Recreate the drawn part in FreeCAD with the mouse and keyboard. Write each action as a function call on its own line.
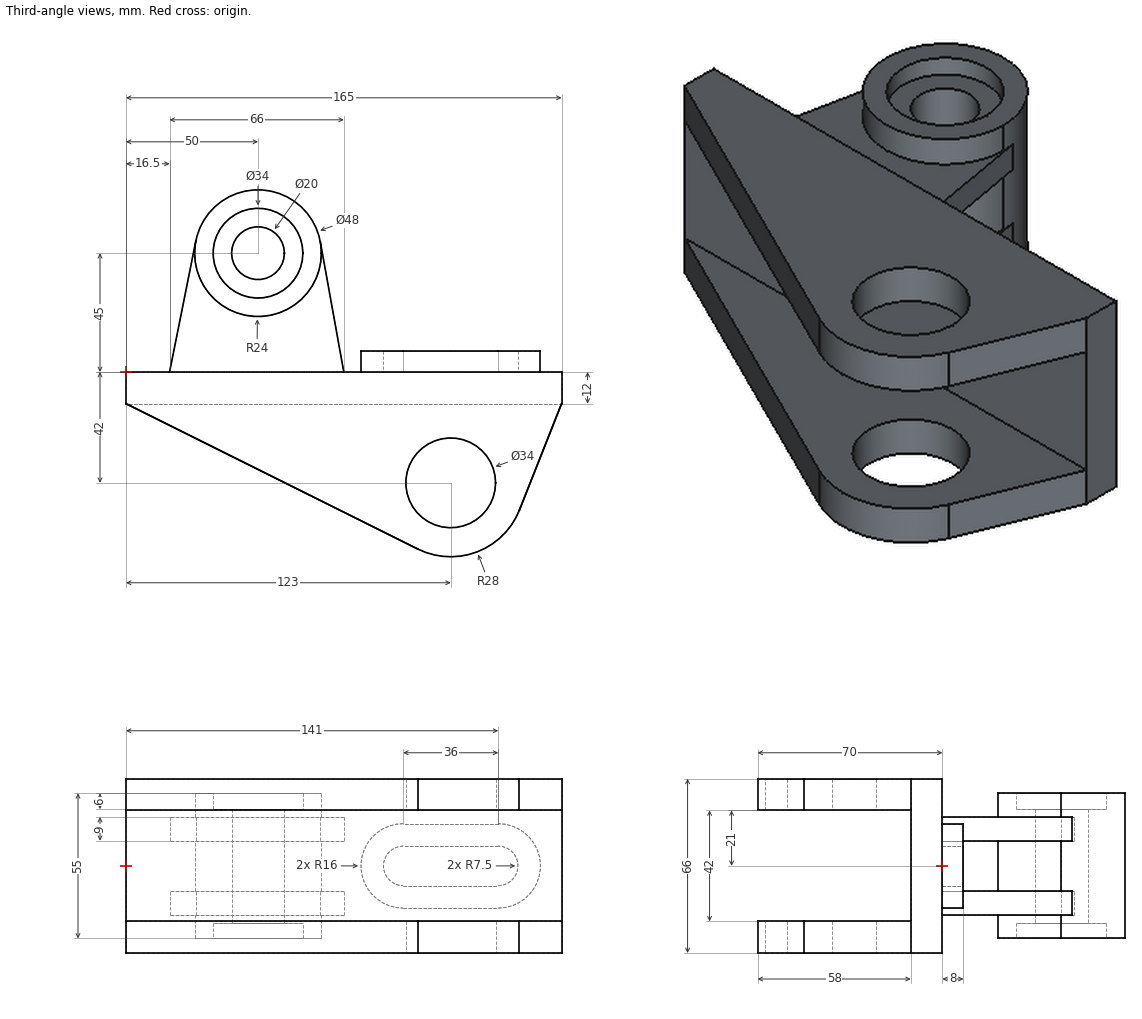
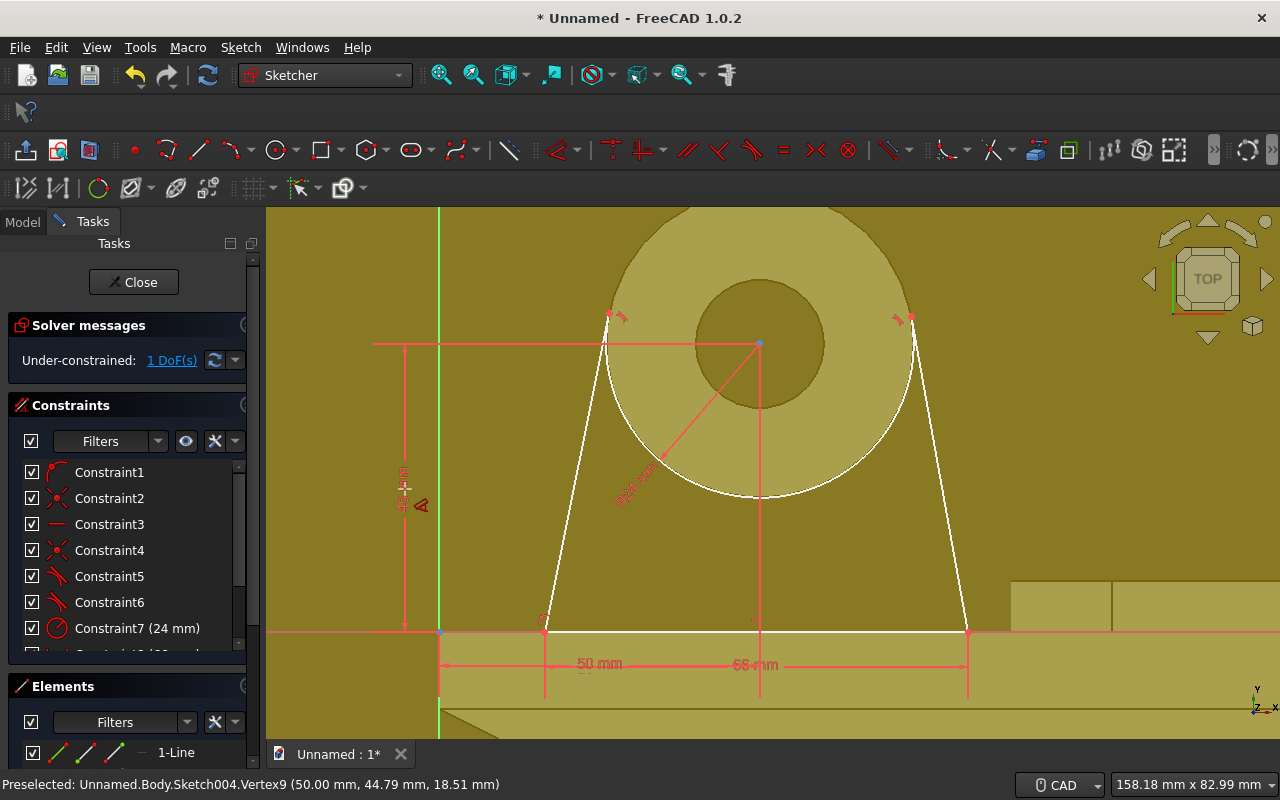
click(545, 632)
click(492, 666)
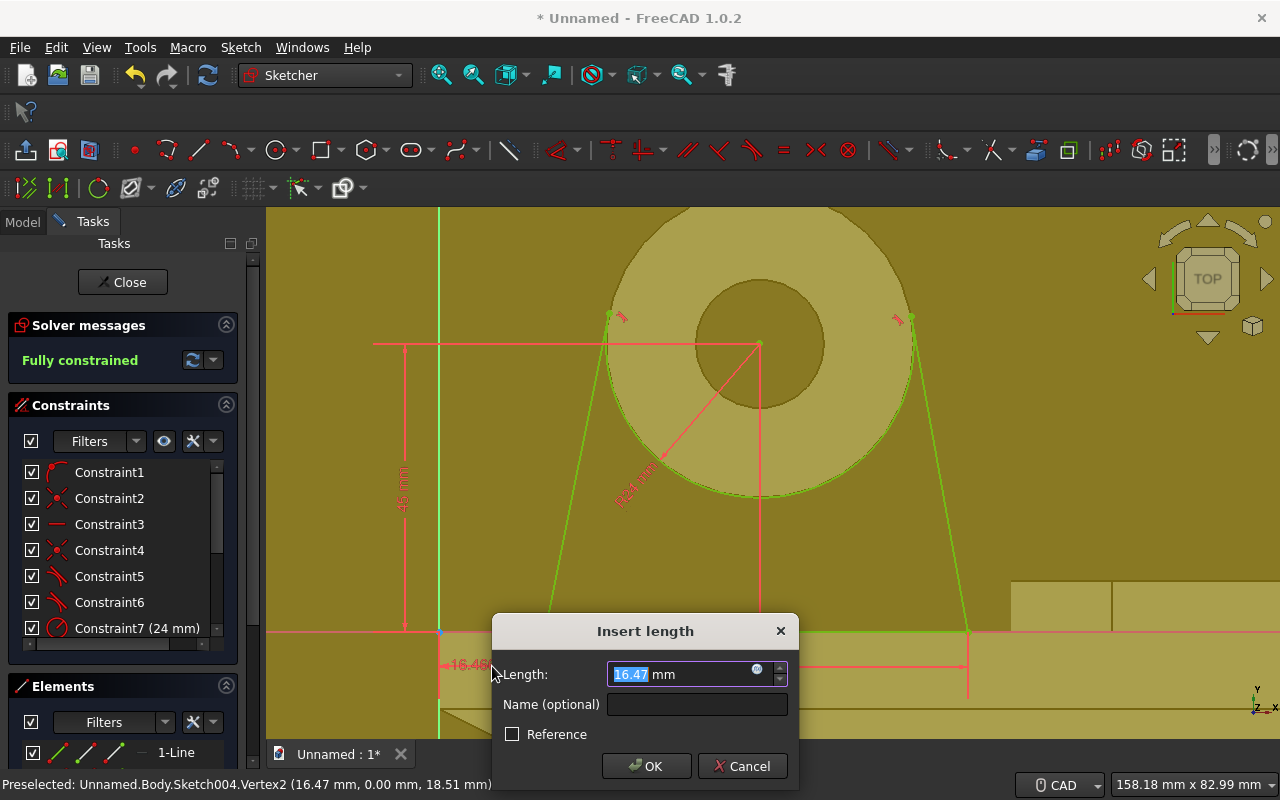
text(16.5)
key(Return)
key(Escape)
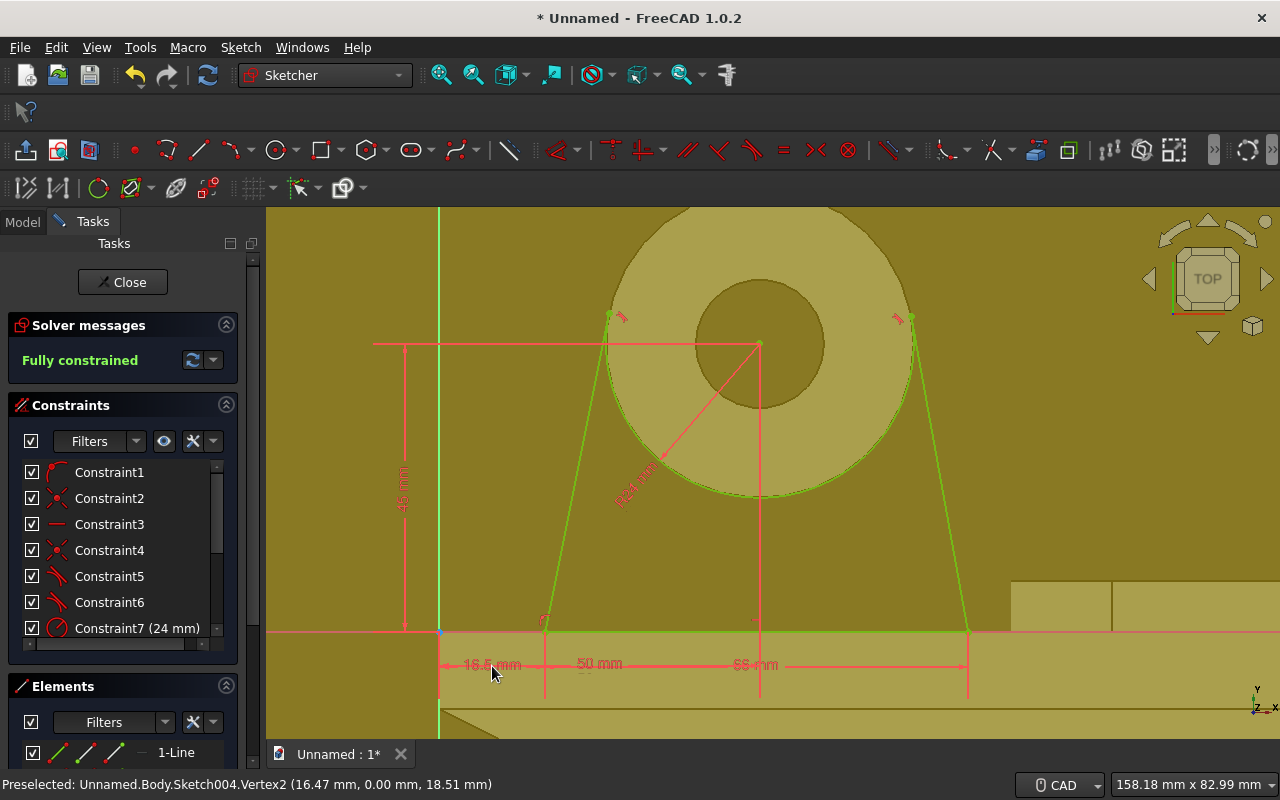
click(123, 282)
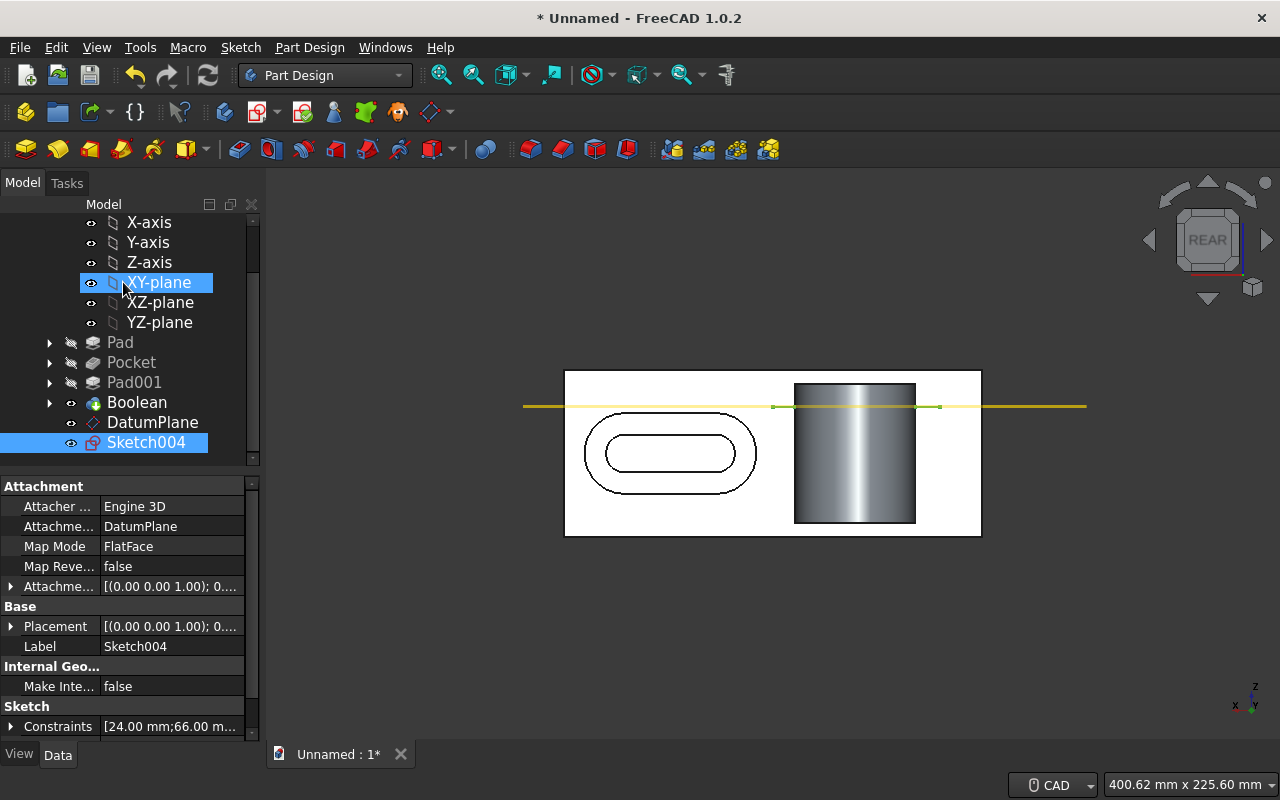
click(26, 150)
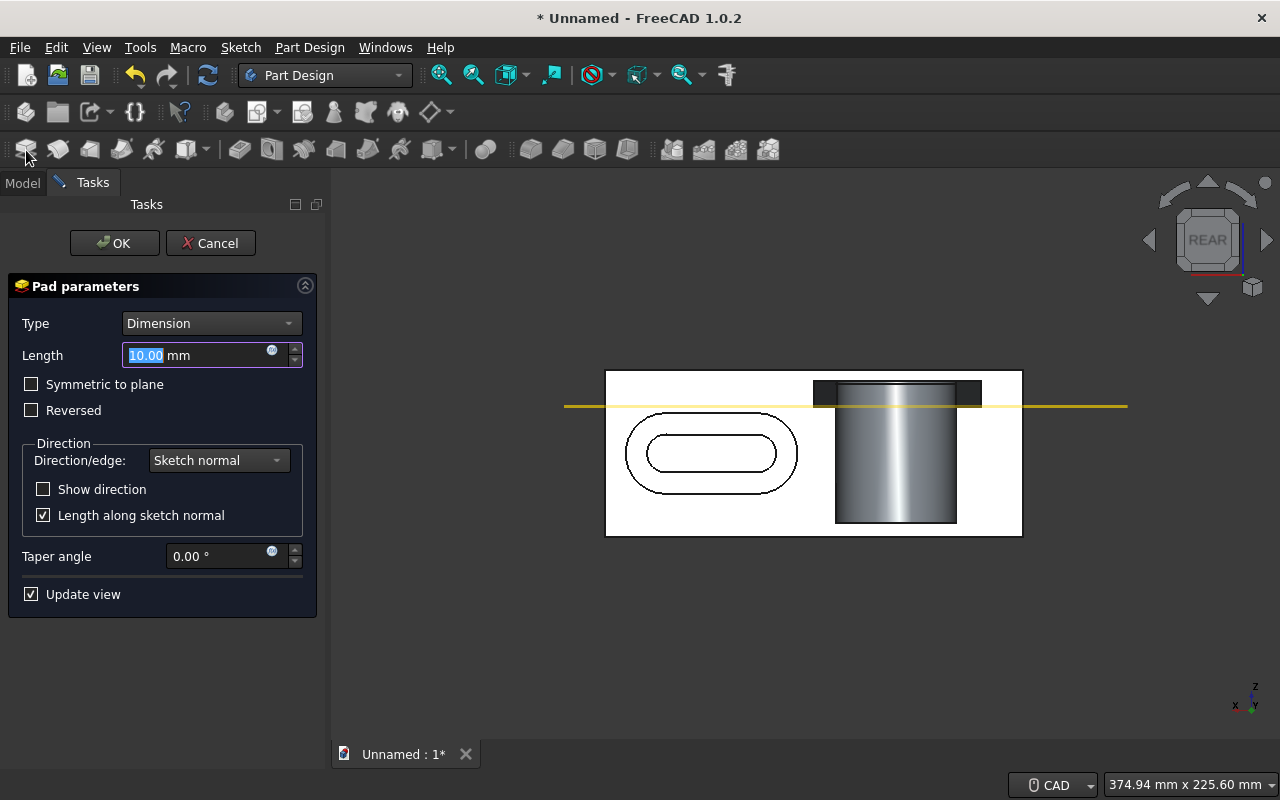
text(9)
key(Tab)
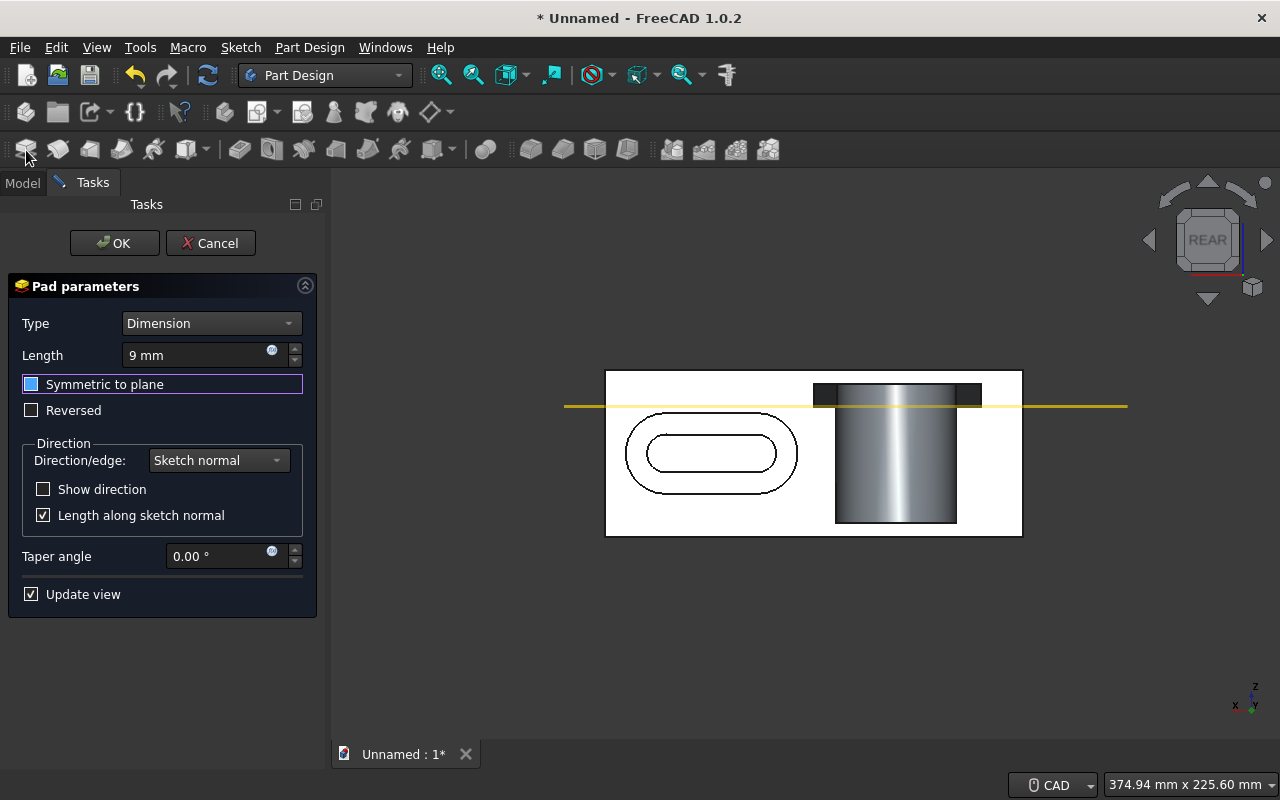
click(30, 410)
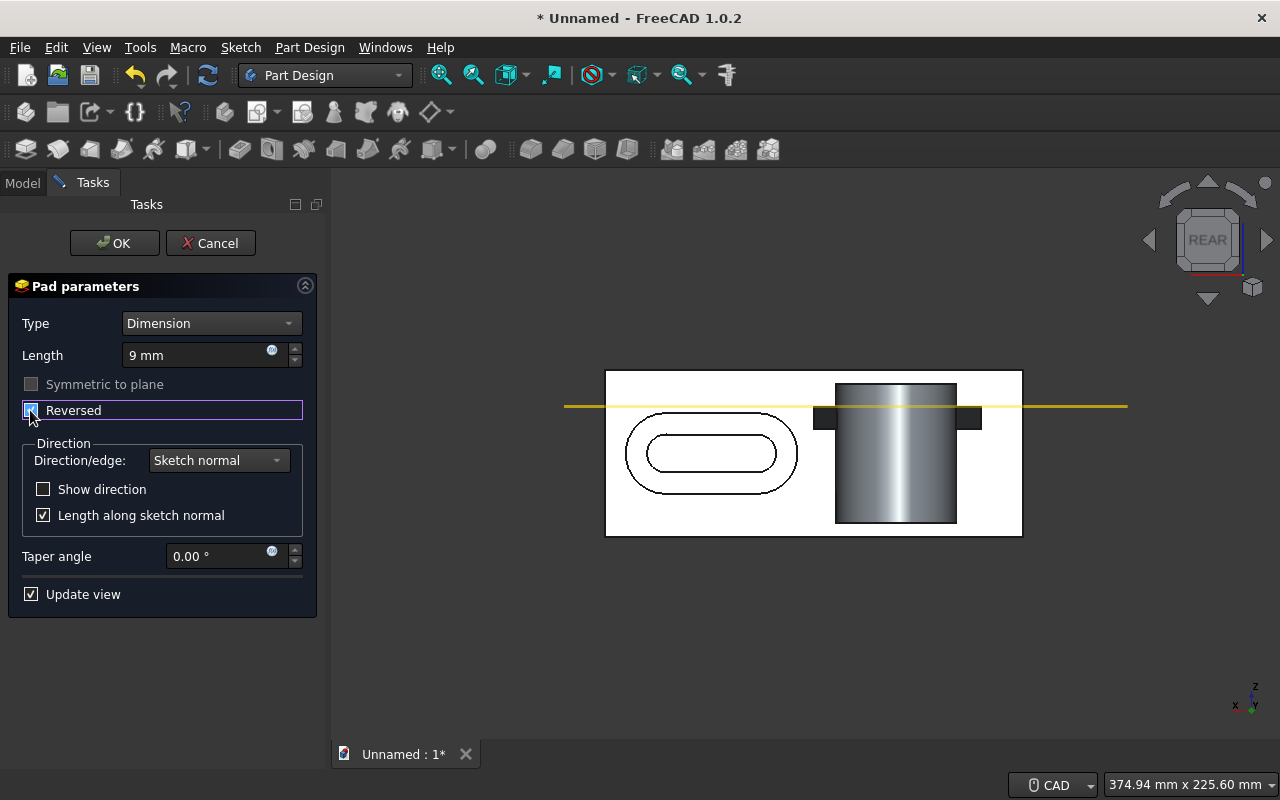
click(115, 243)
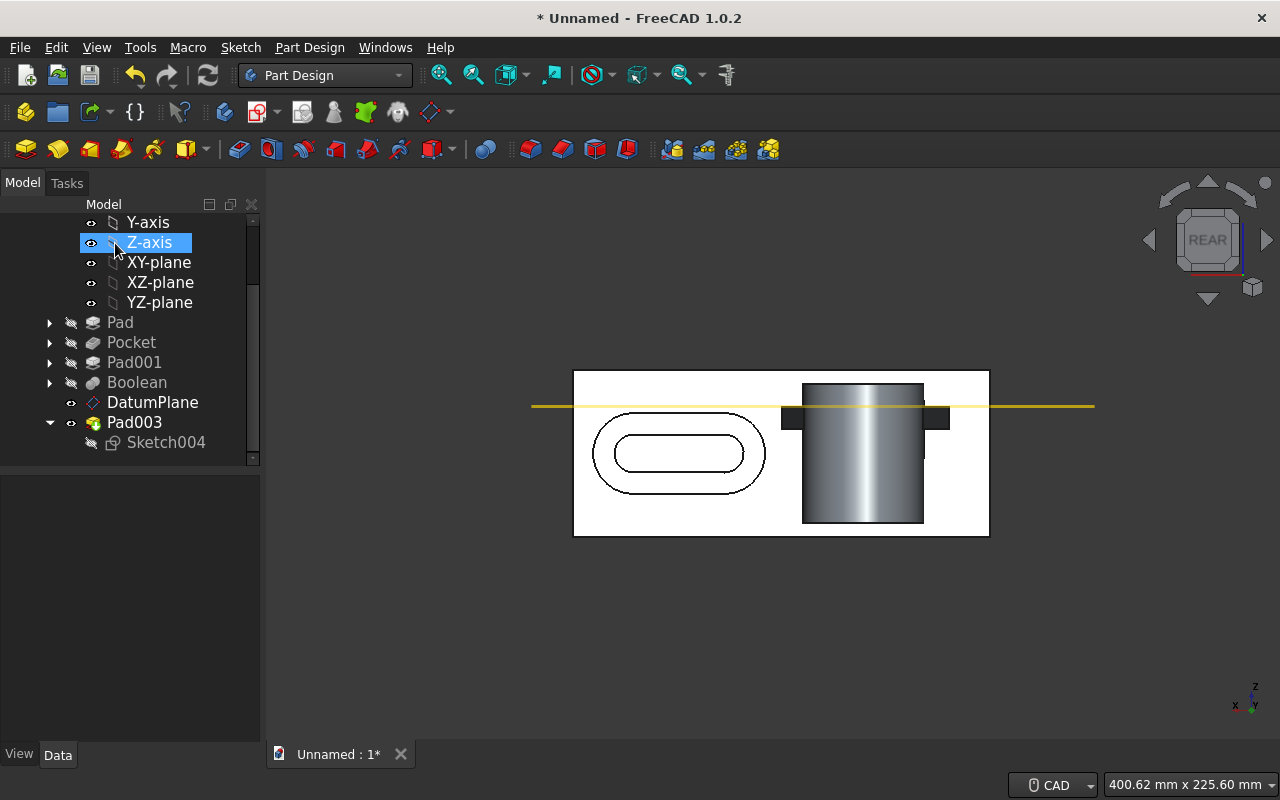
click(116, 403)
key(space)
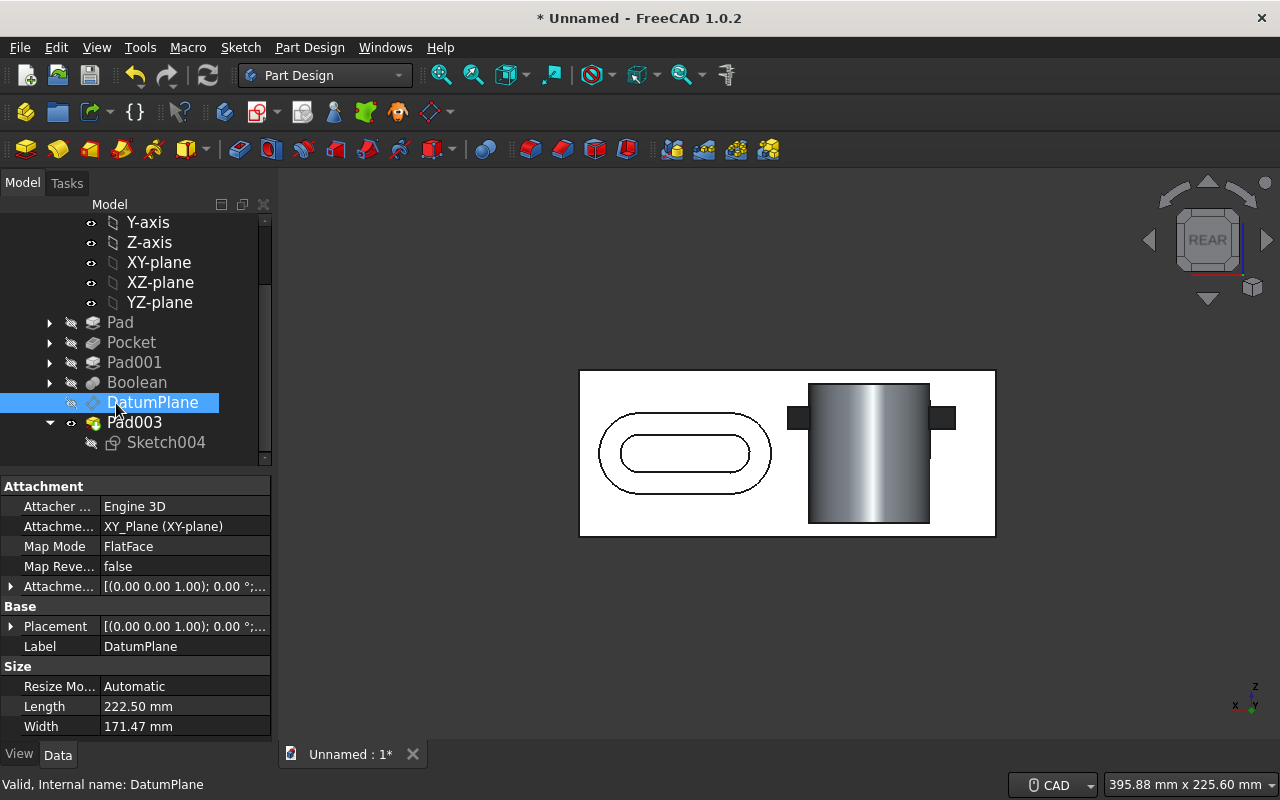
key(v)
key(f)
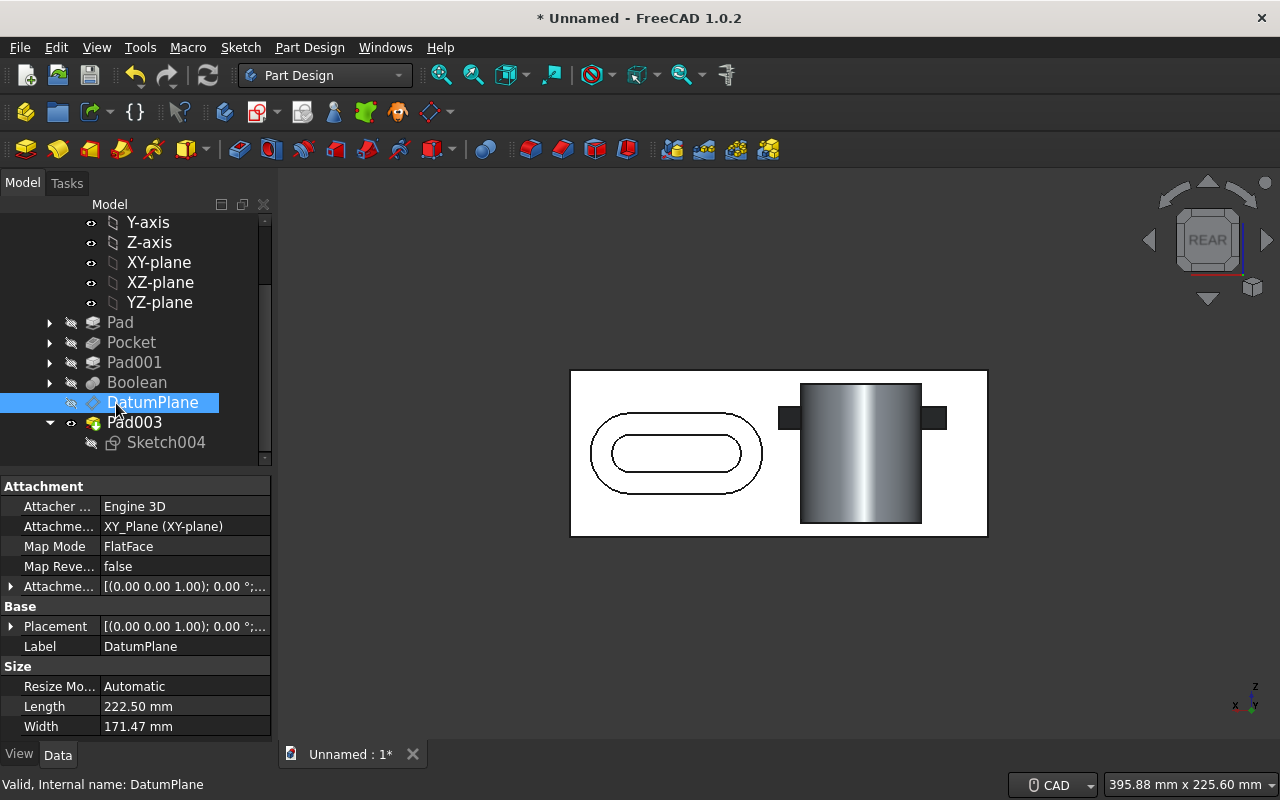
click(116, 423)